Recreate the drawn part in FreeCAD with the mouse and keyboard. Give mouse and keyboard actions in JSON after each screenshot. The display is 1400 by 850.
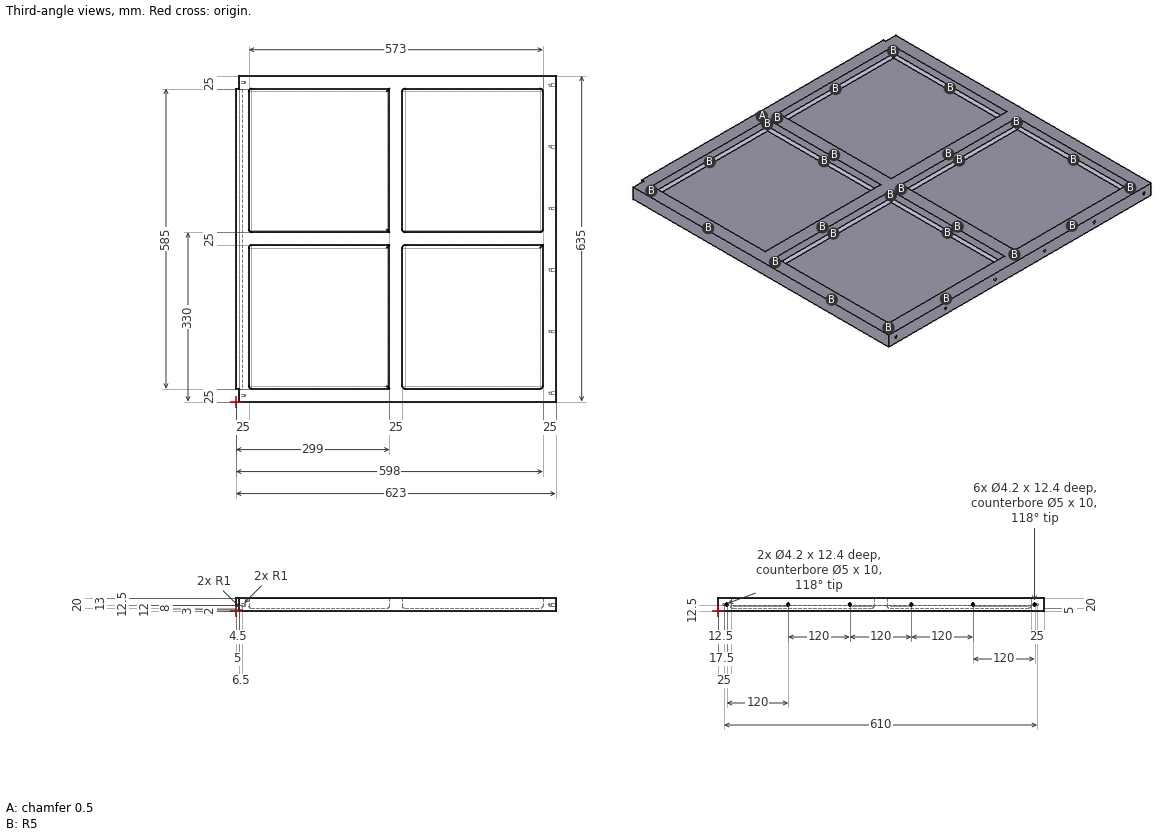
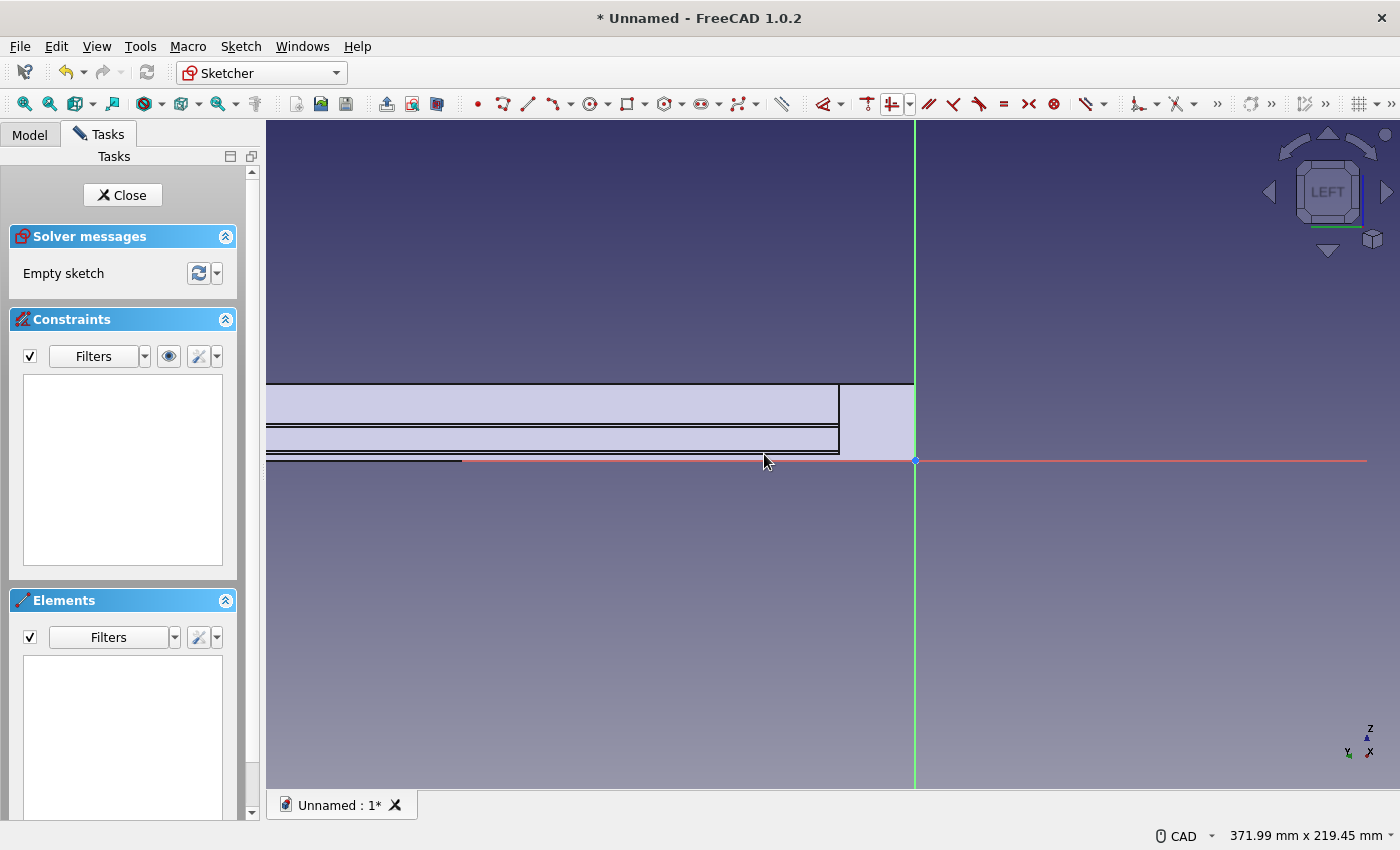
{"action": "scroll", "coordinate": [1231, 464], "scroll_direction": "down", "scroll_amount": 5}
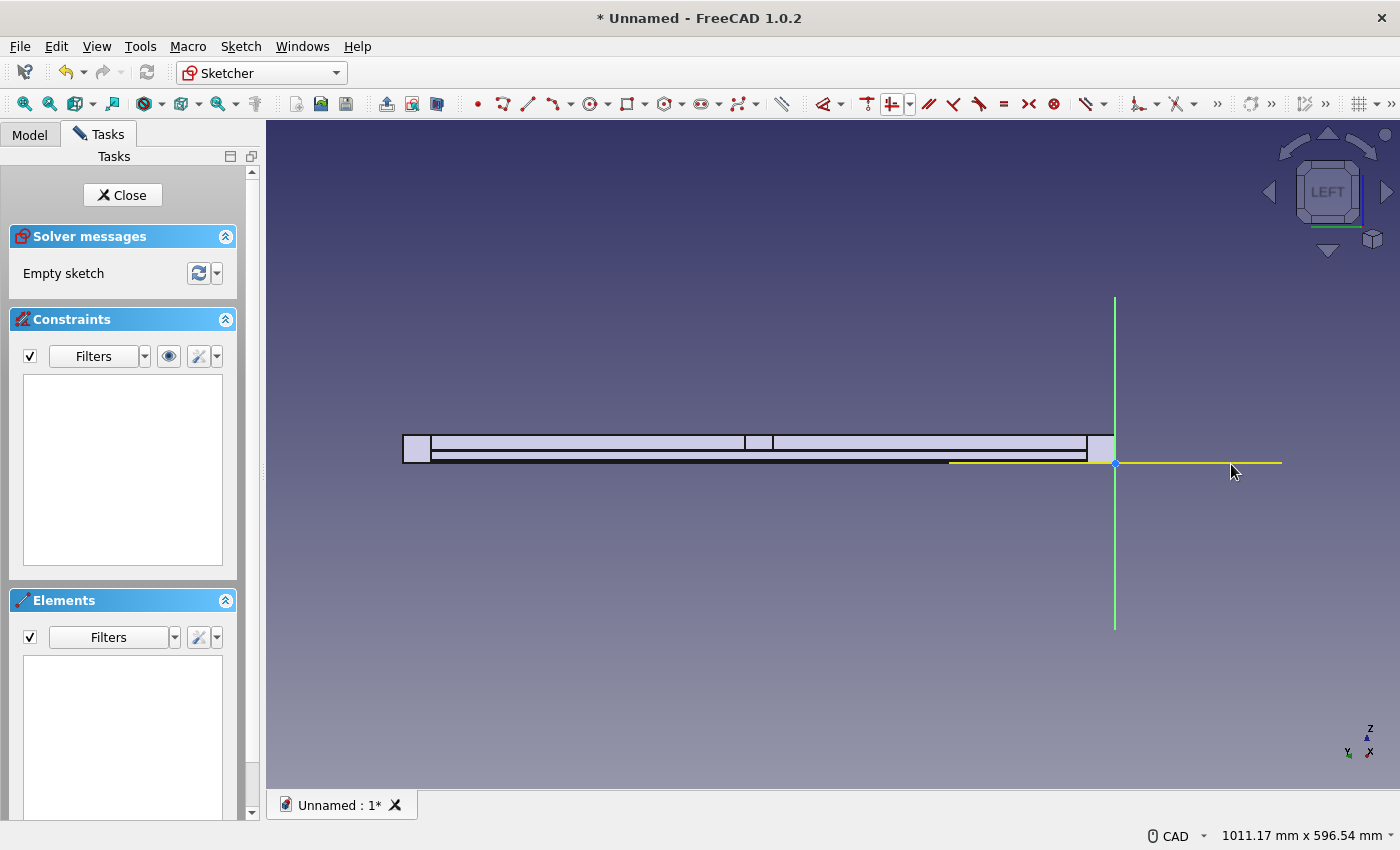
{"action": "left_click", "coordinate": [590, 104]}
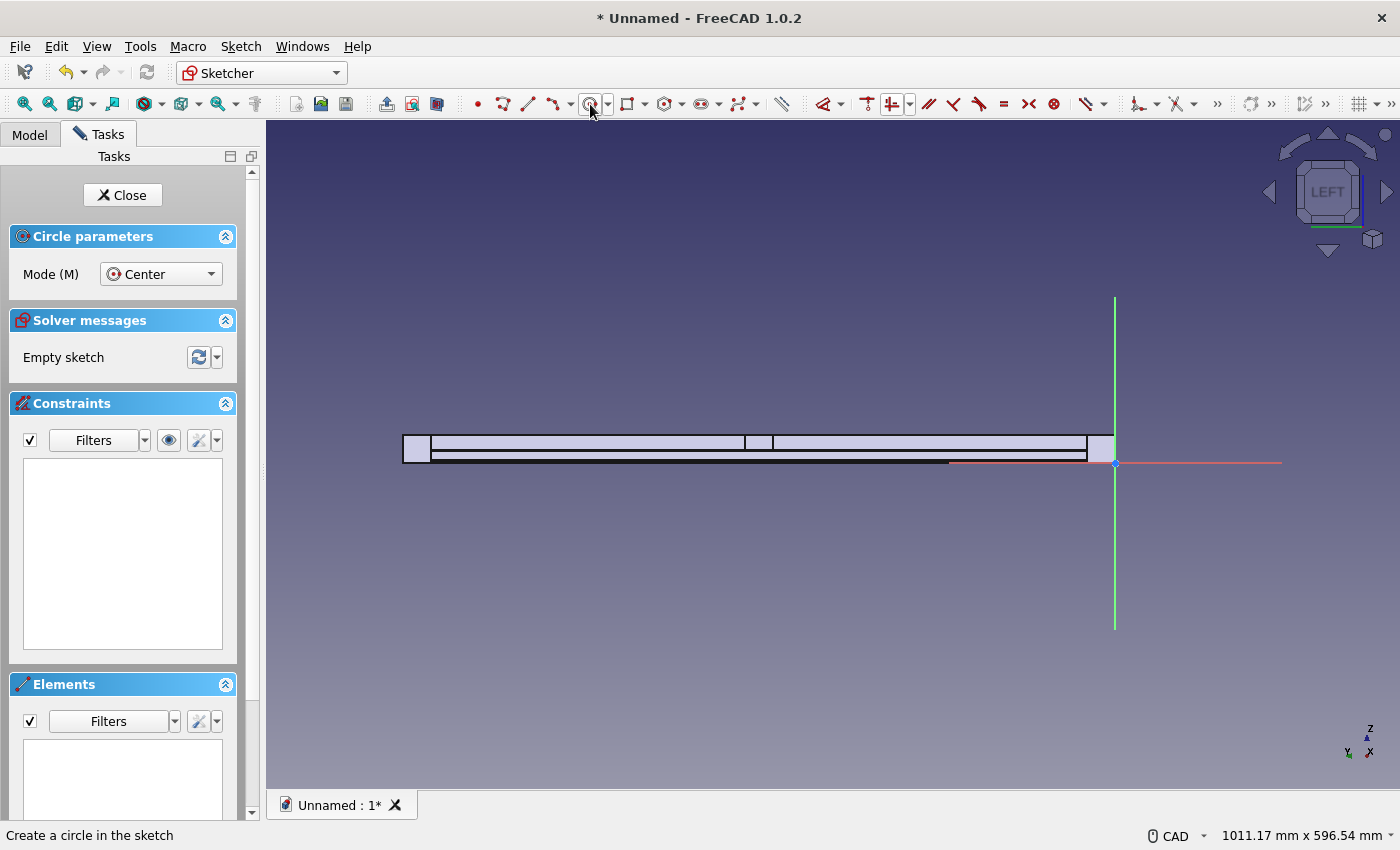
{"action": "scroll", "coordinate": [1101, 449], "scroll_direction": "up", "scroll_amount": 12}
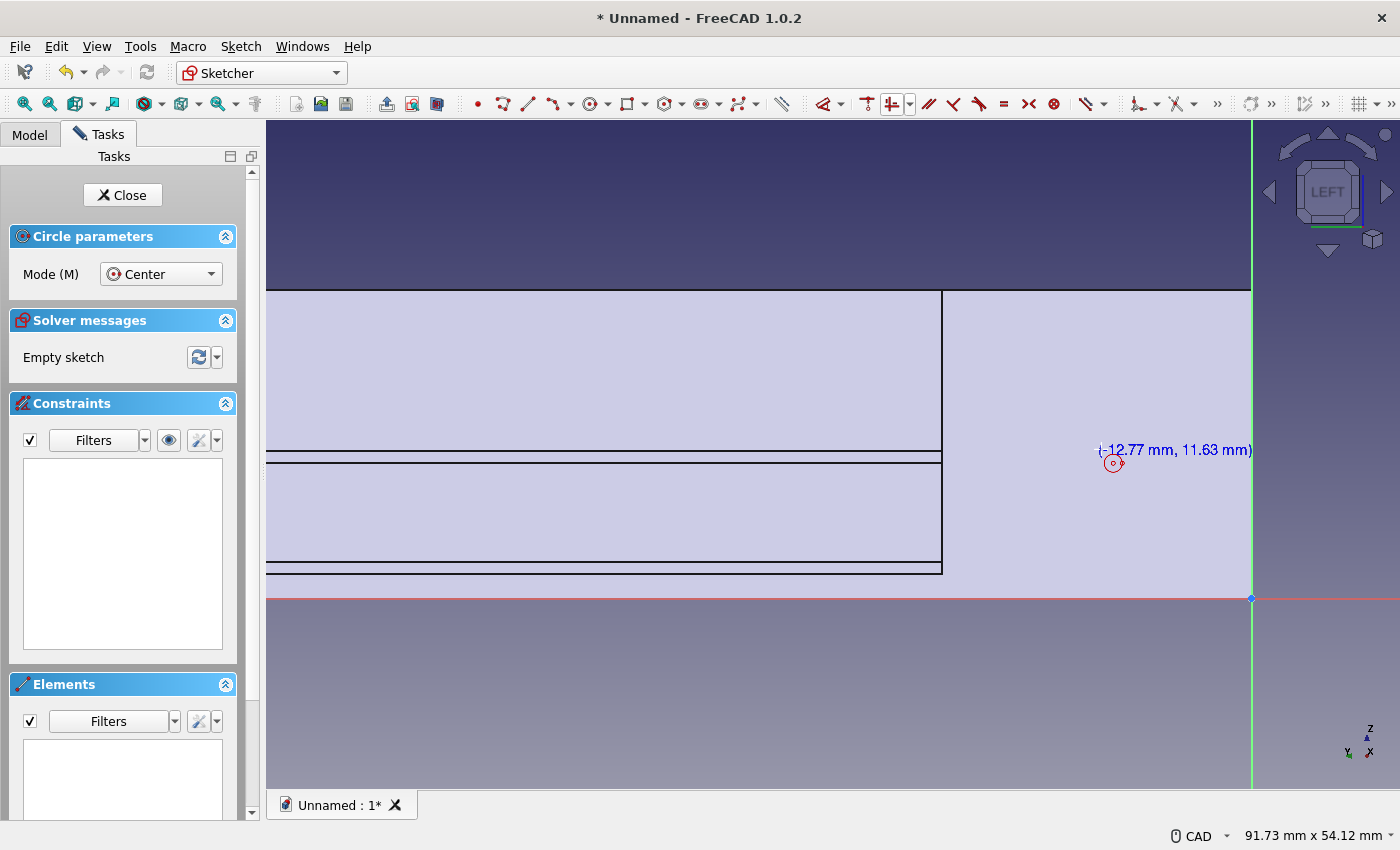
{"action": "scroll", "coordinate": [1101, 449], "scroll_direction": "down", "scroll_amount": 12}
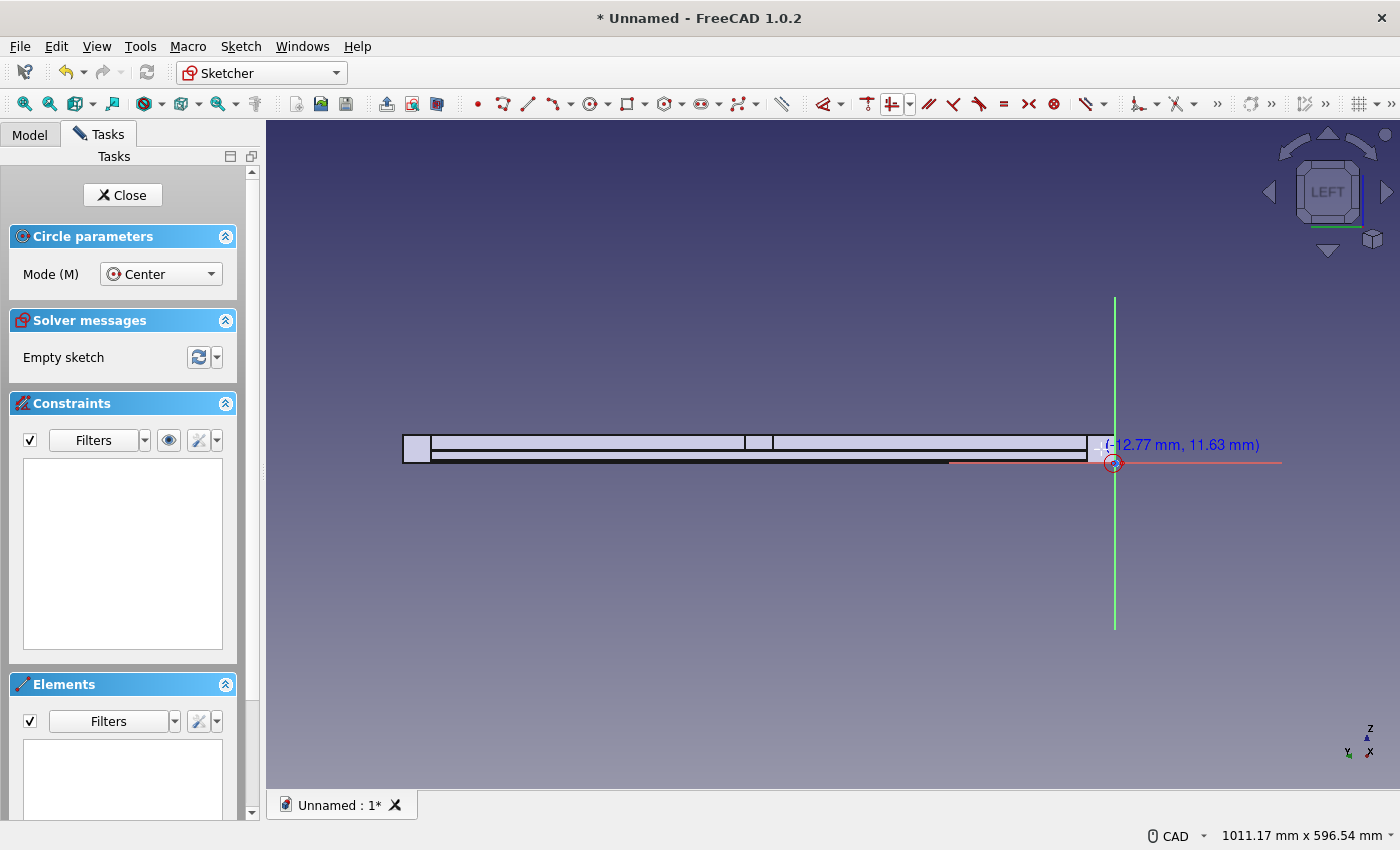
{"action": "left_click", "coordinate": [1101, 449]}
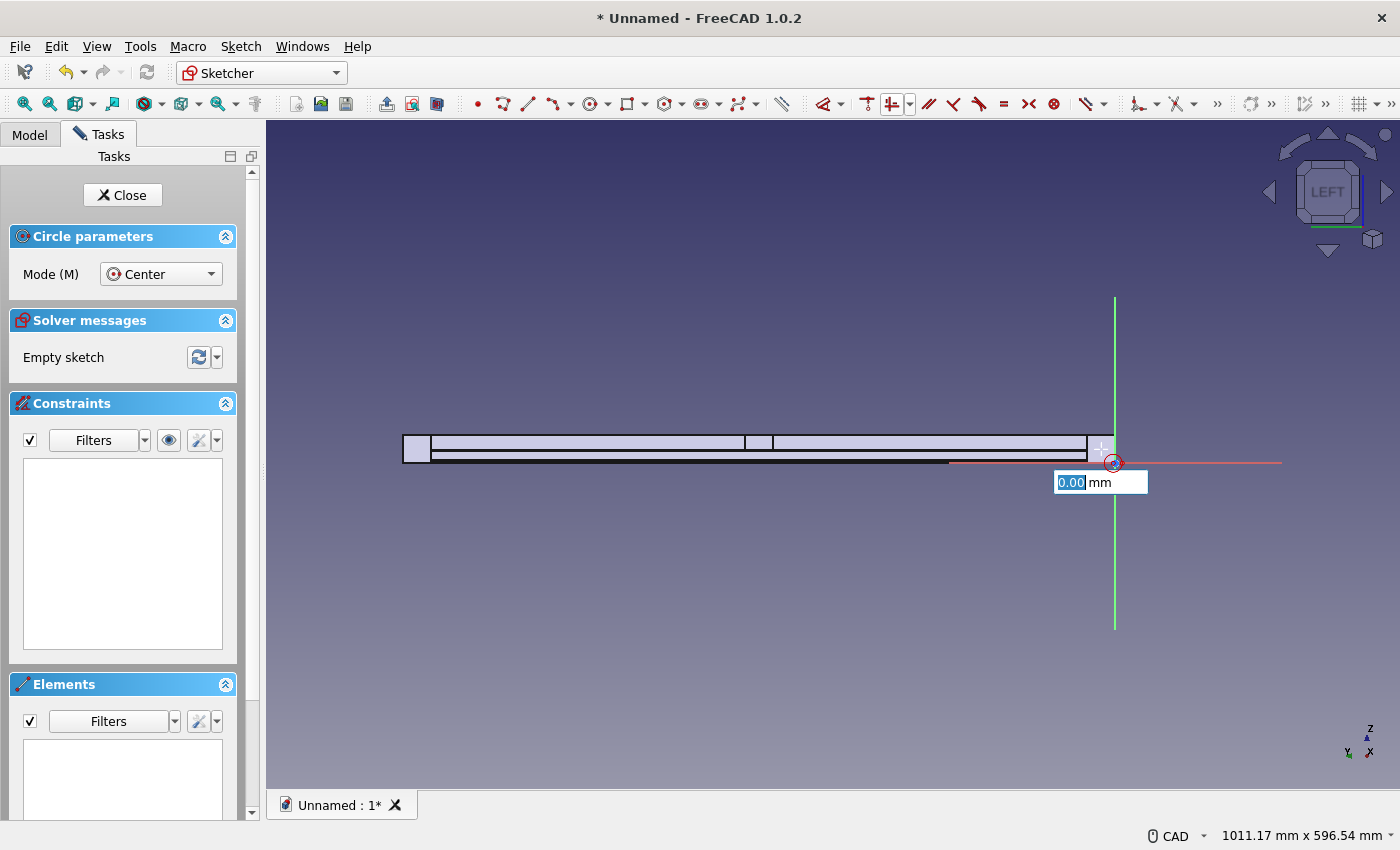
{"action": "scroll", "coordinate": [1100, 447], "scroll_direction": "up", "scroll_amount": 10}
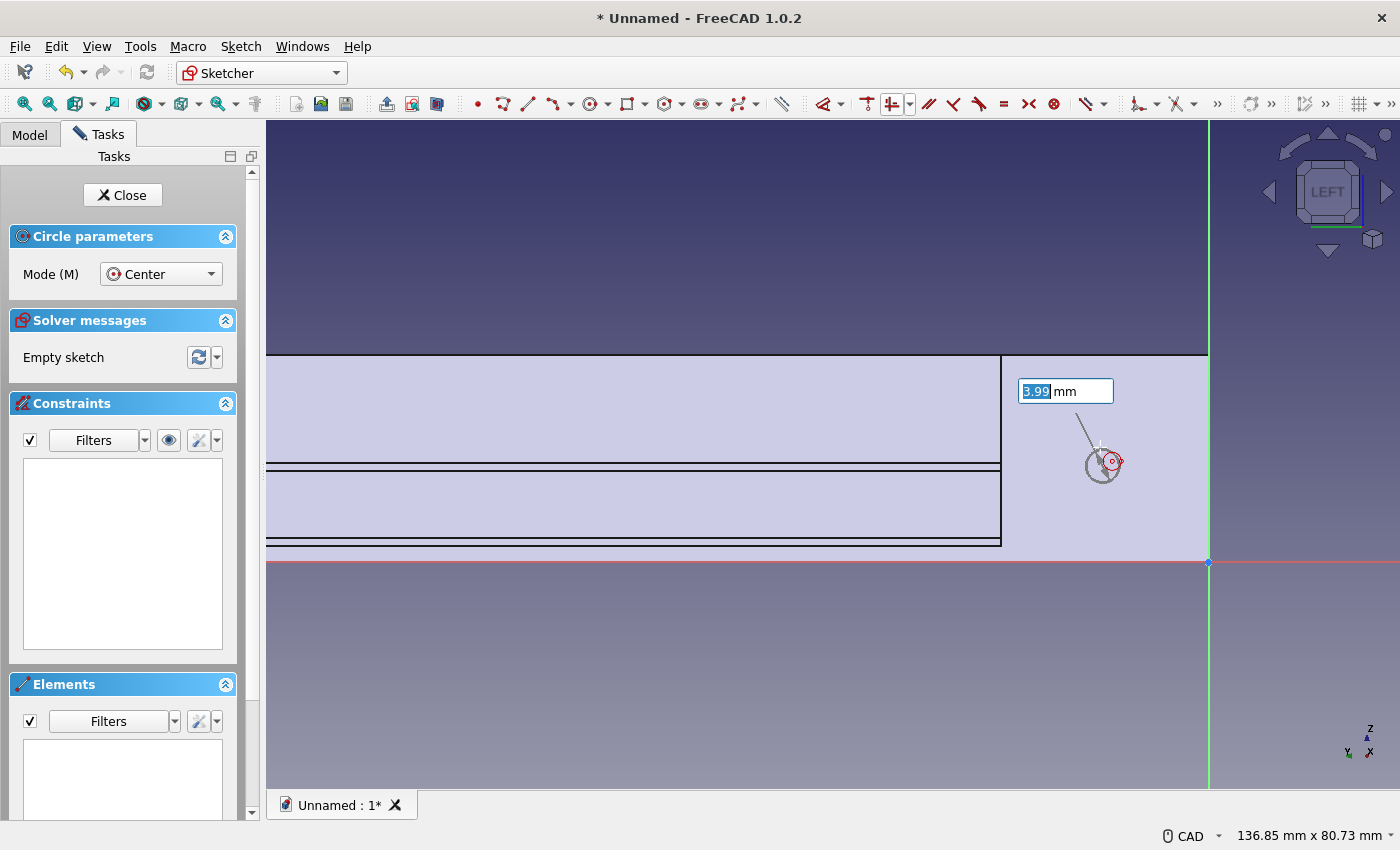
{"action": "left_click", "coordinate": [1093, 447]}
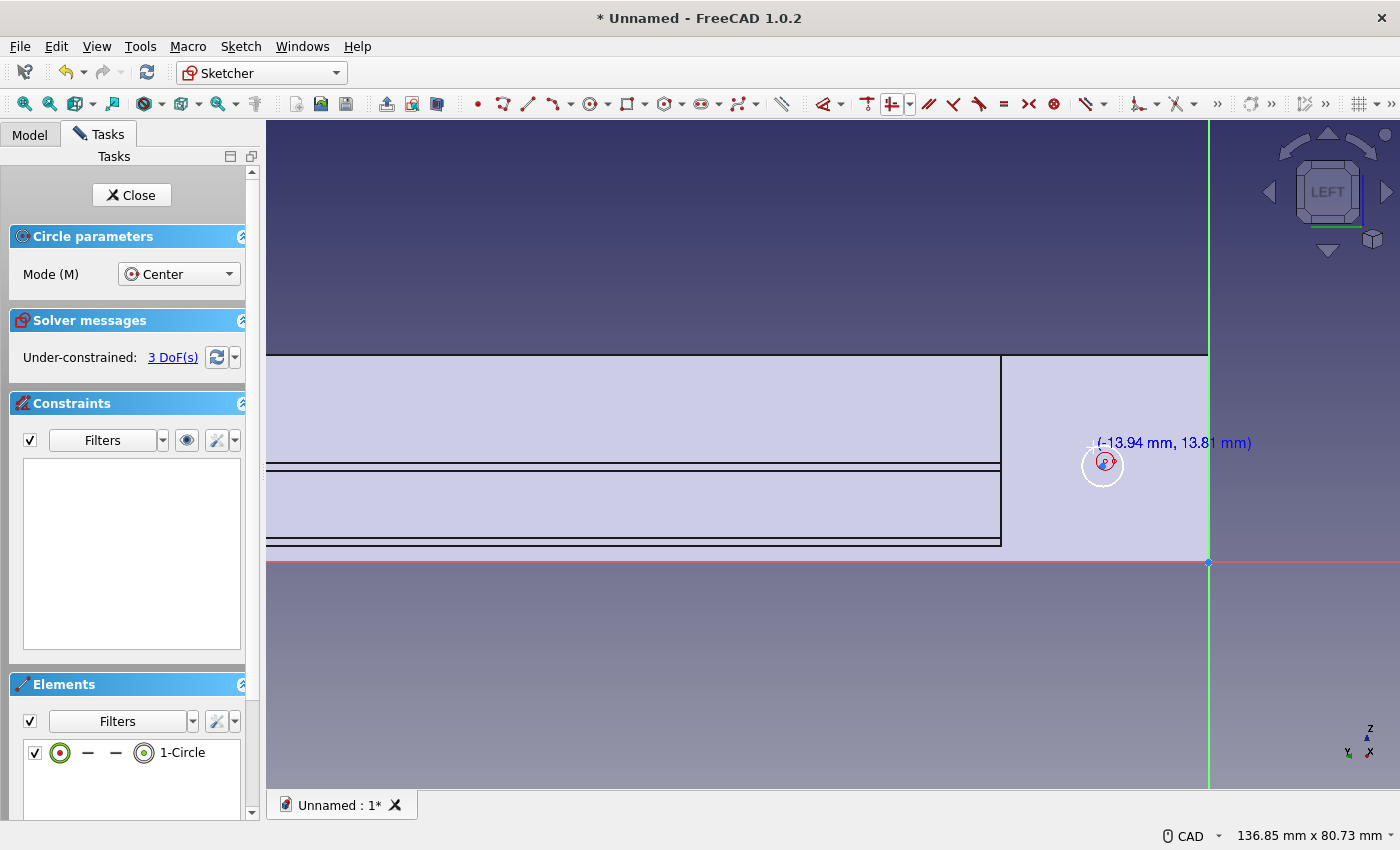
{"action": "scroll", "coordinate": [1100, 447], "scroll_direction": "down", "scroll_amount": 10}